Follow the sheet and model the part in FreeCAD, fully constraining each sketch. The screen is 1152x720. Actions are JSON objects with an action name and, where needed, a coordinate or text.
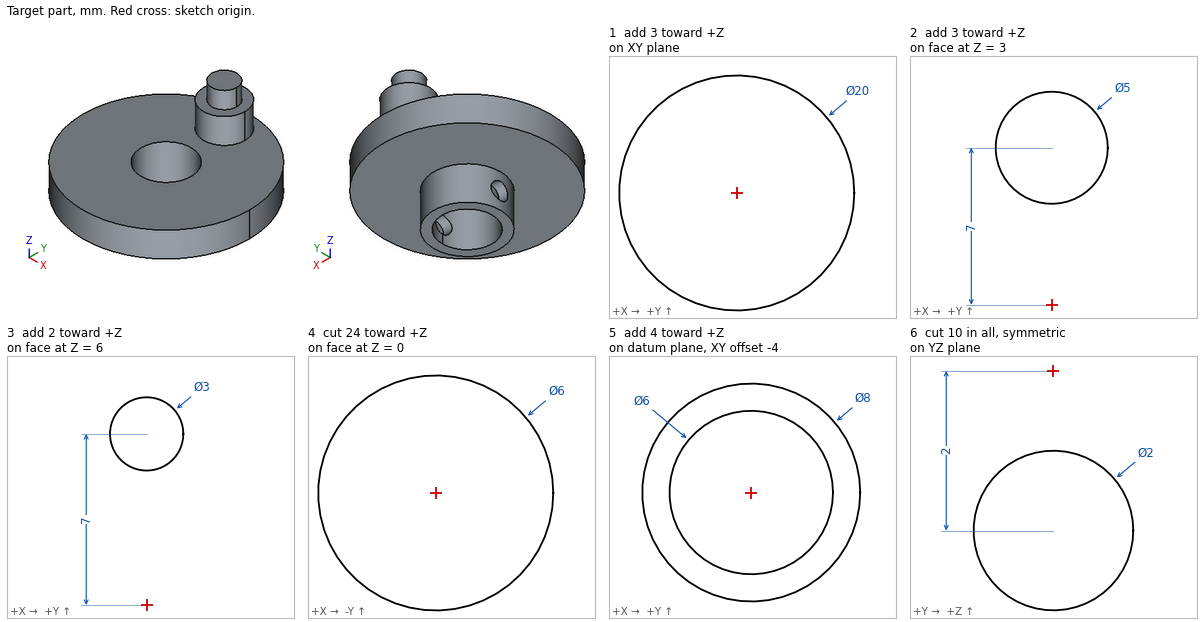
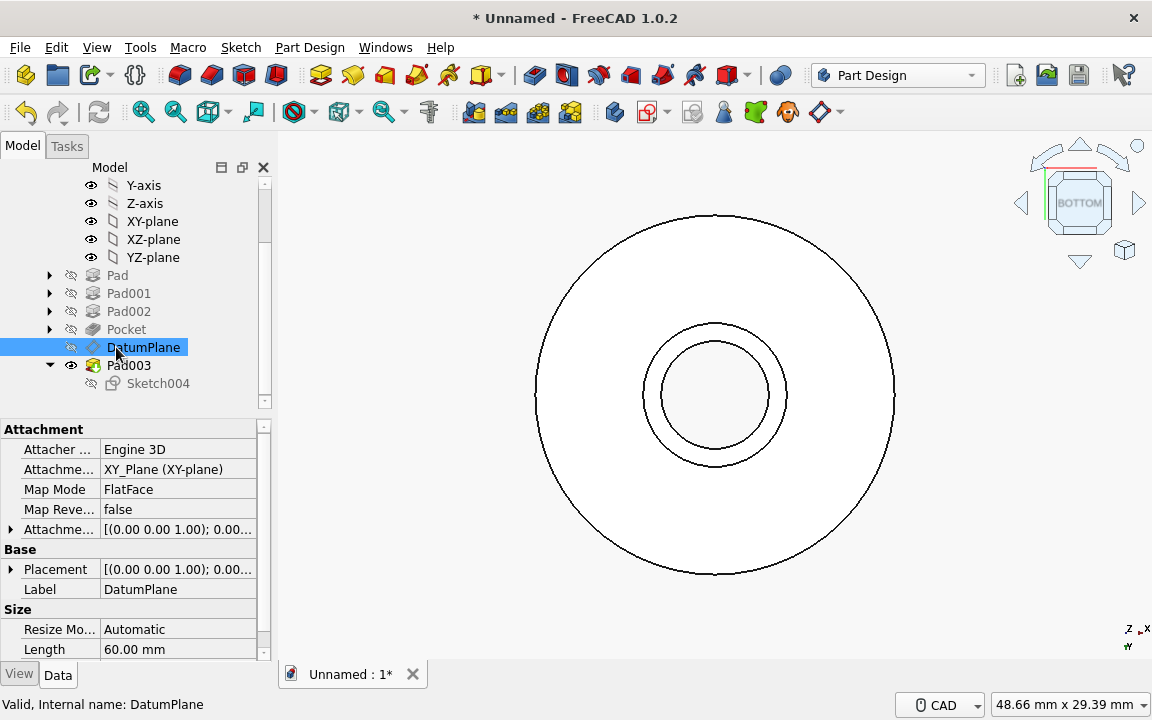
{"action": "left_click", "coordinate": [318, 619]}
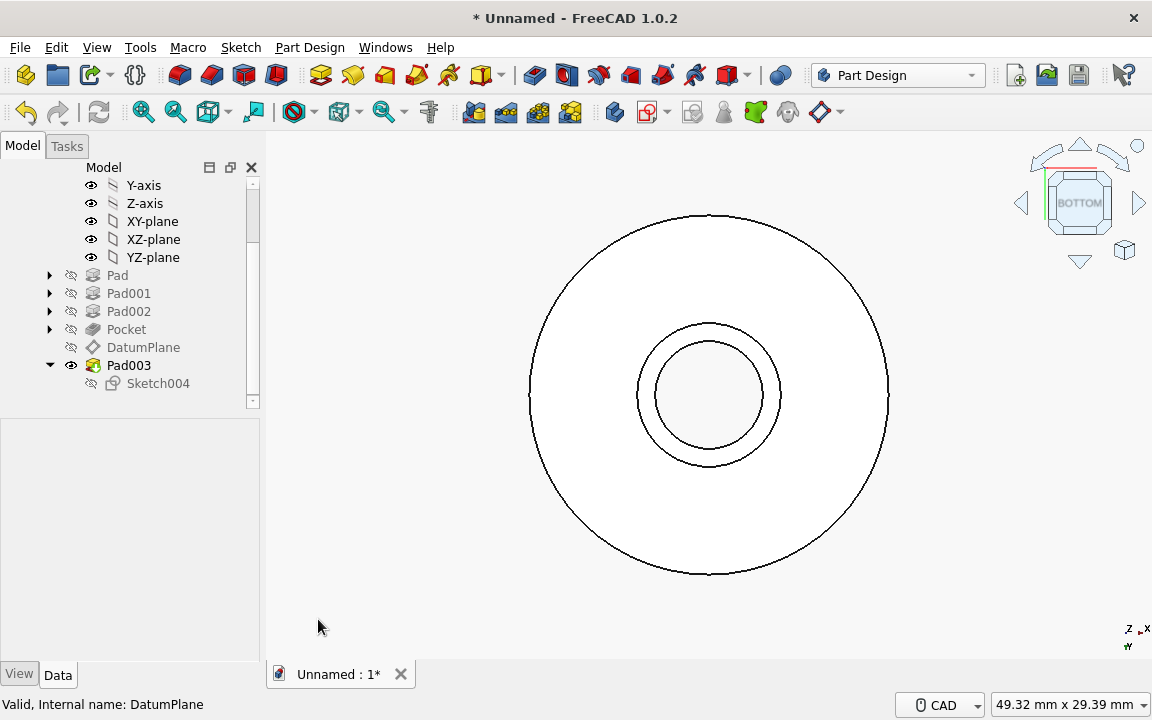
{"action": "left_click", "coordinate": [648, 112]}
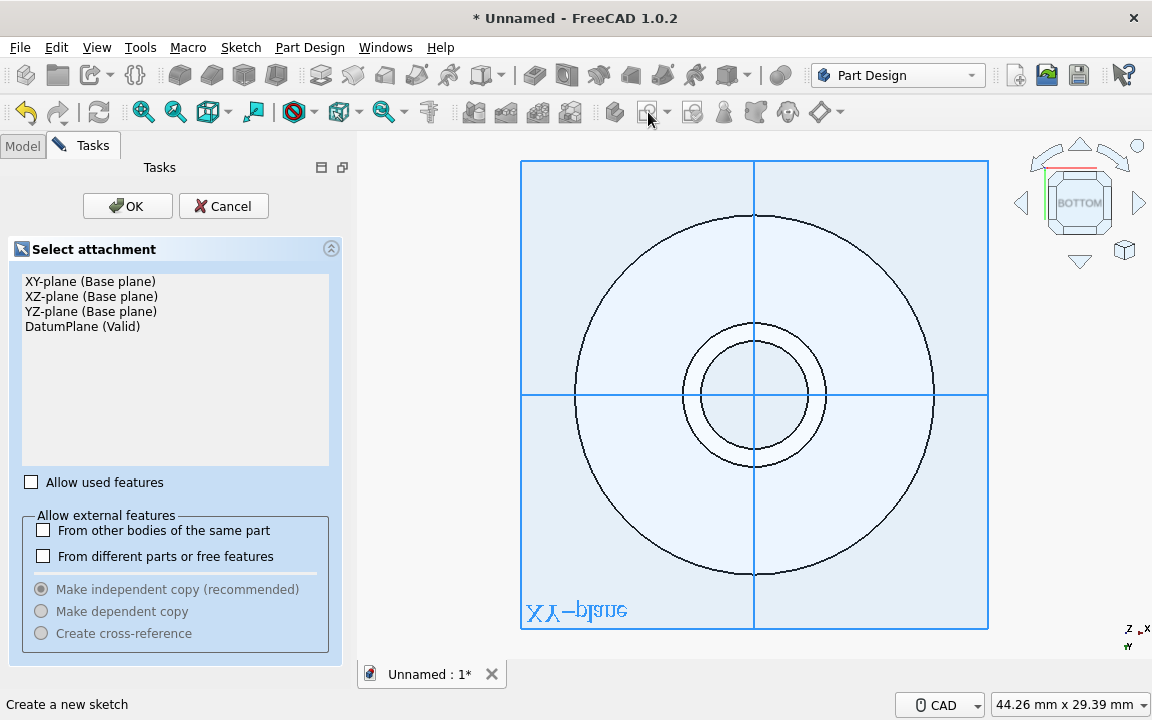
{"action": "left_click", "coordinate": [82, 312]}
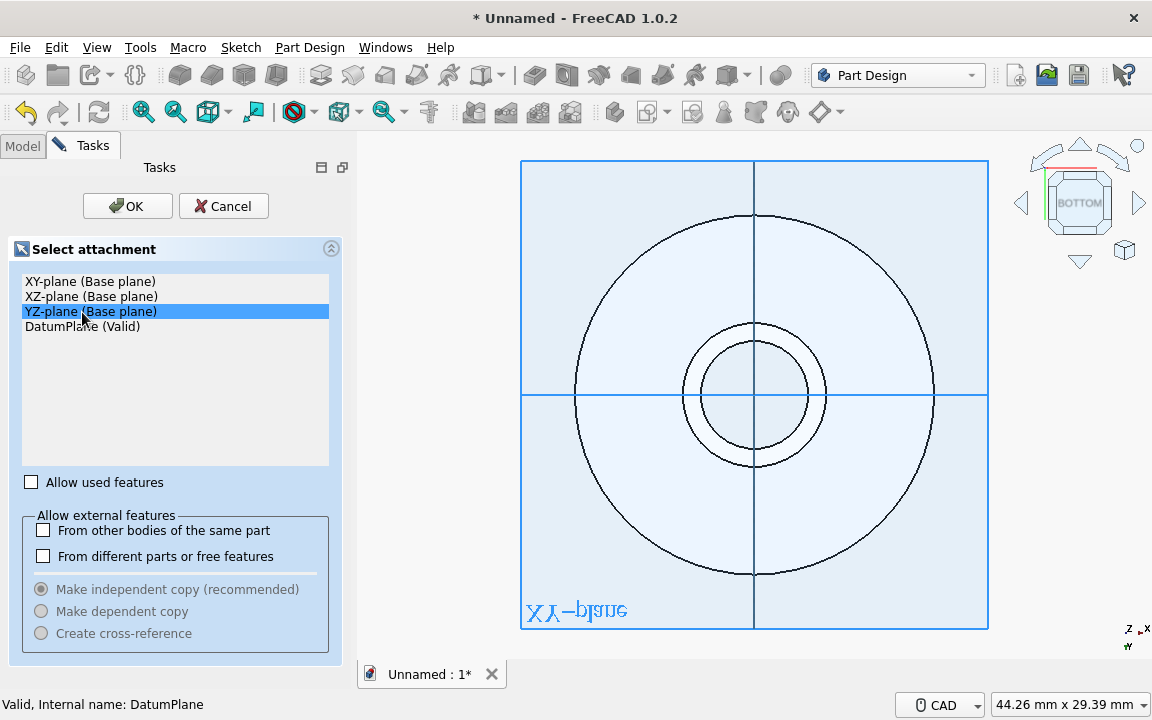
{"action": "left_click", "coordinate": [128, 206]}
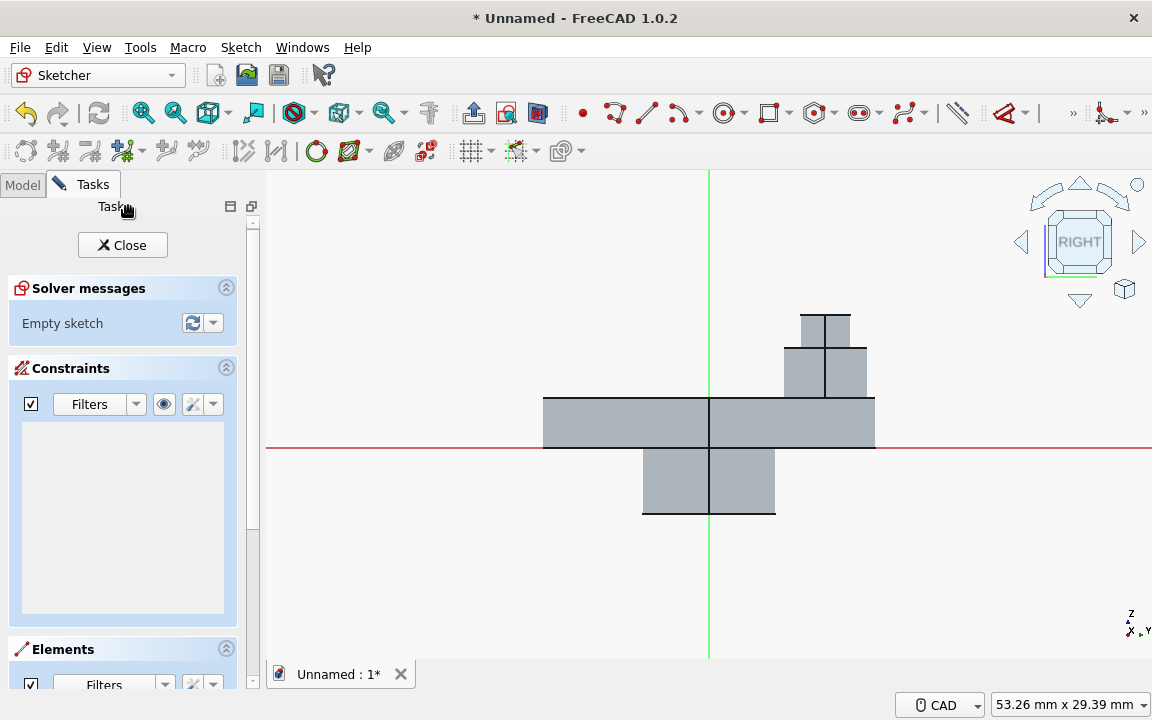
{"action": "key", "text": "q s"}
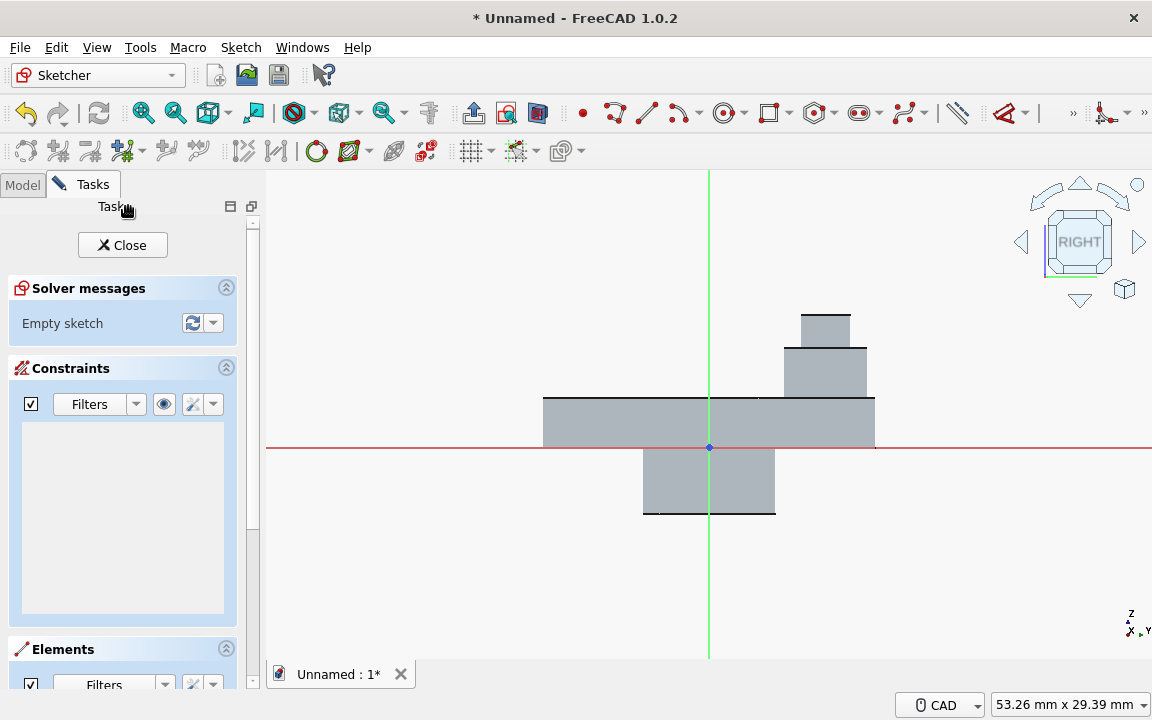
{"action": "scroll", "coordinate": [723, 484], "scroll_direction": "up", "scroll_amount": 9}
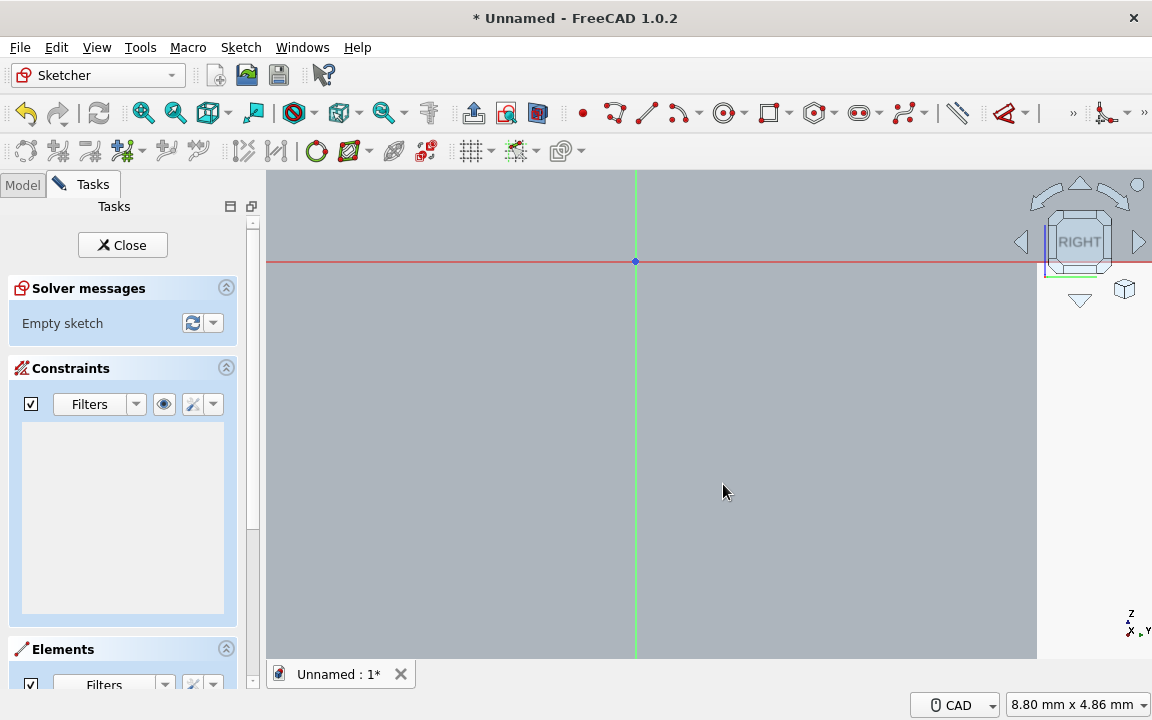
{"action": "left_click", "coordinate": [724, 114]}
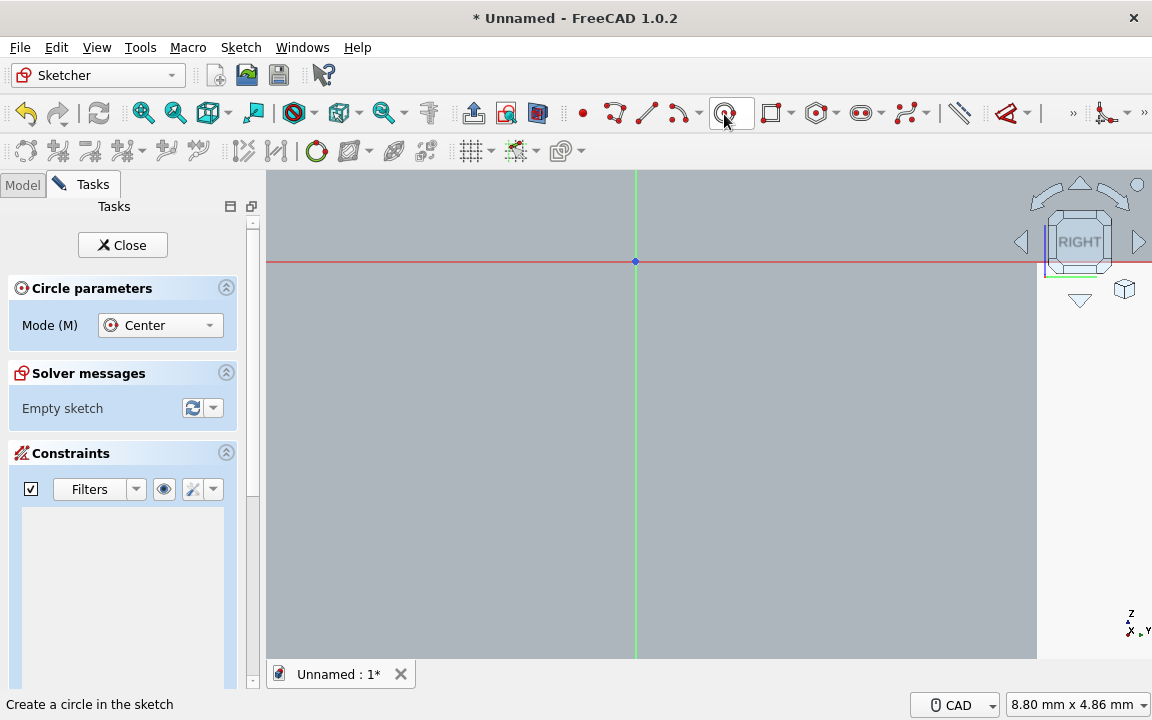
{"action": "left_click", "coordinate": [636, 463]}
{"action": "left_click", "coordinate": [707, 392]}
{"action": "key", "text": "Escape"}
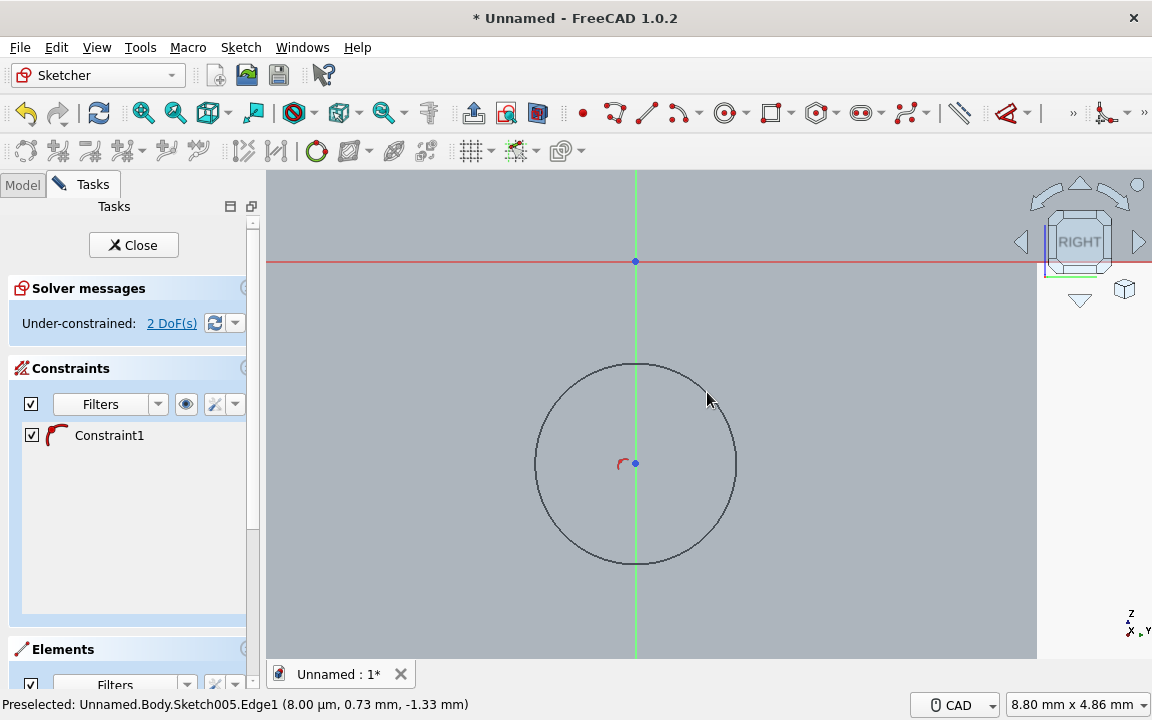
{"action": "left_click", "coordinate": [1006, 114]}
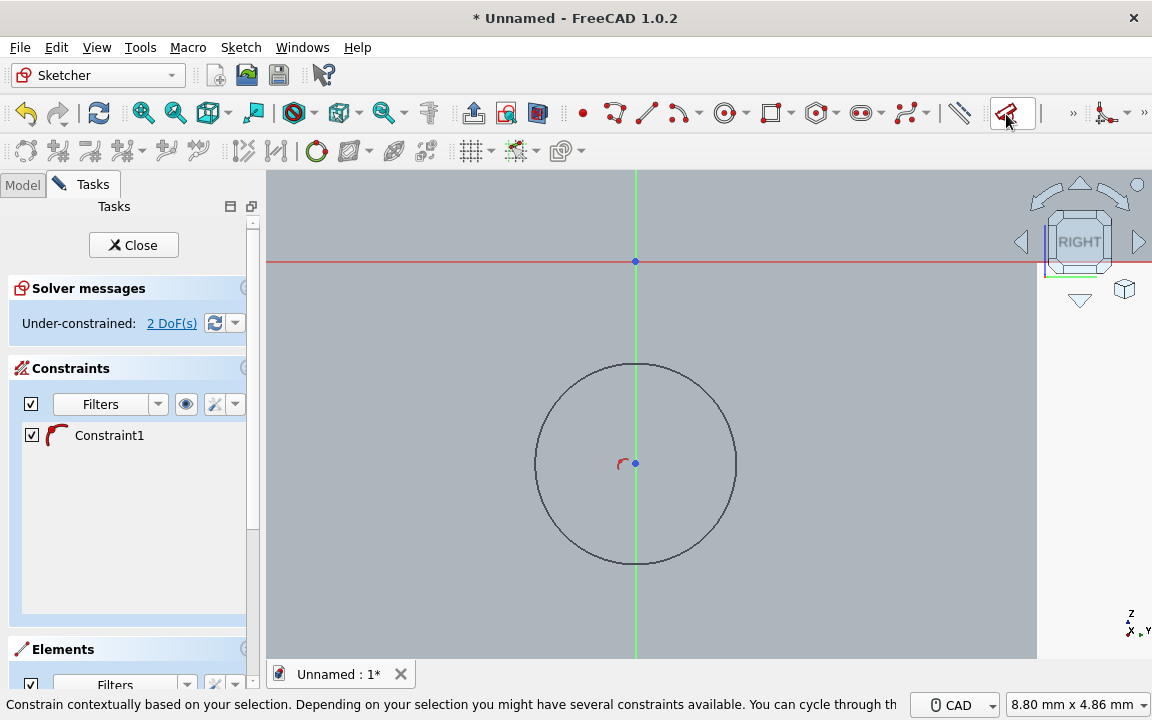
{"action": "left_click", "coordinate": [707, 393]}
{"action": "left_click", "coordinate": [730, 370]}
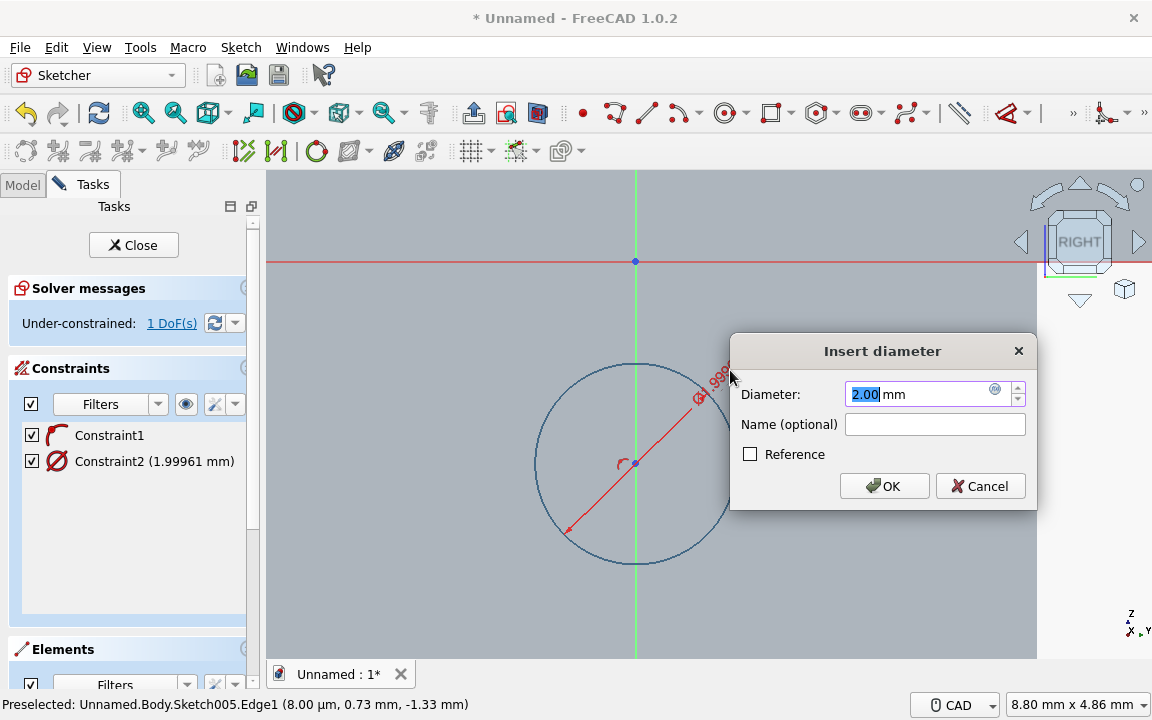
{"action": "type", "text": "2"}
{"action": "key", "text": "Return"}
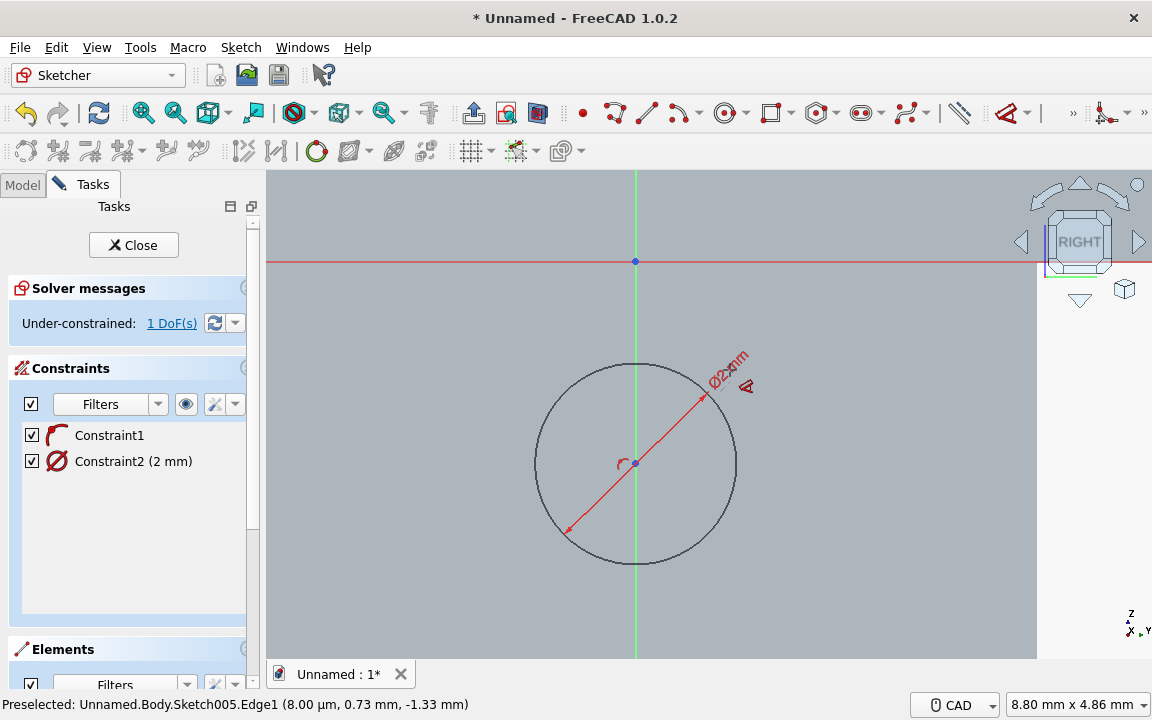
{"action": "left_click", "coordinate": [636, 464]}
{"action": "left_click", "coordinate": [670, 316]}